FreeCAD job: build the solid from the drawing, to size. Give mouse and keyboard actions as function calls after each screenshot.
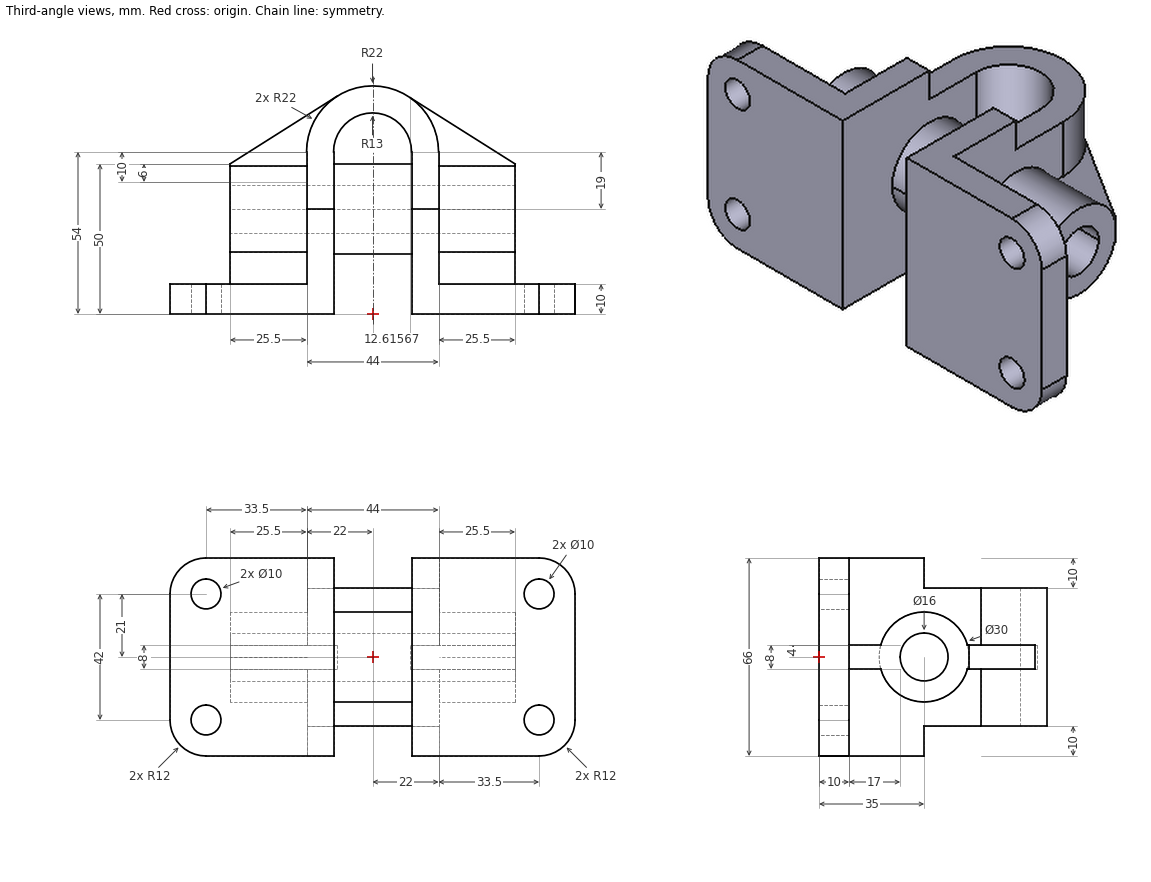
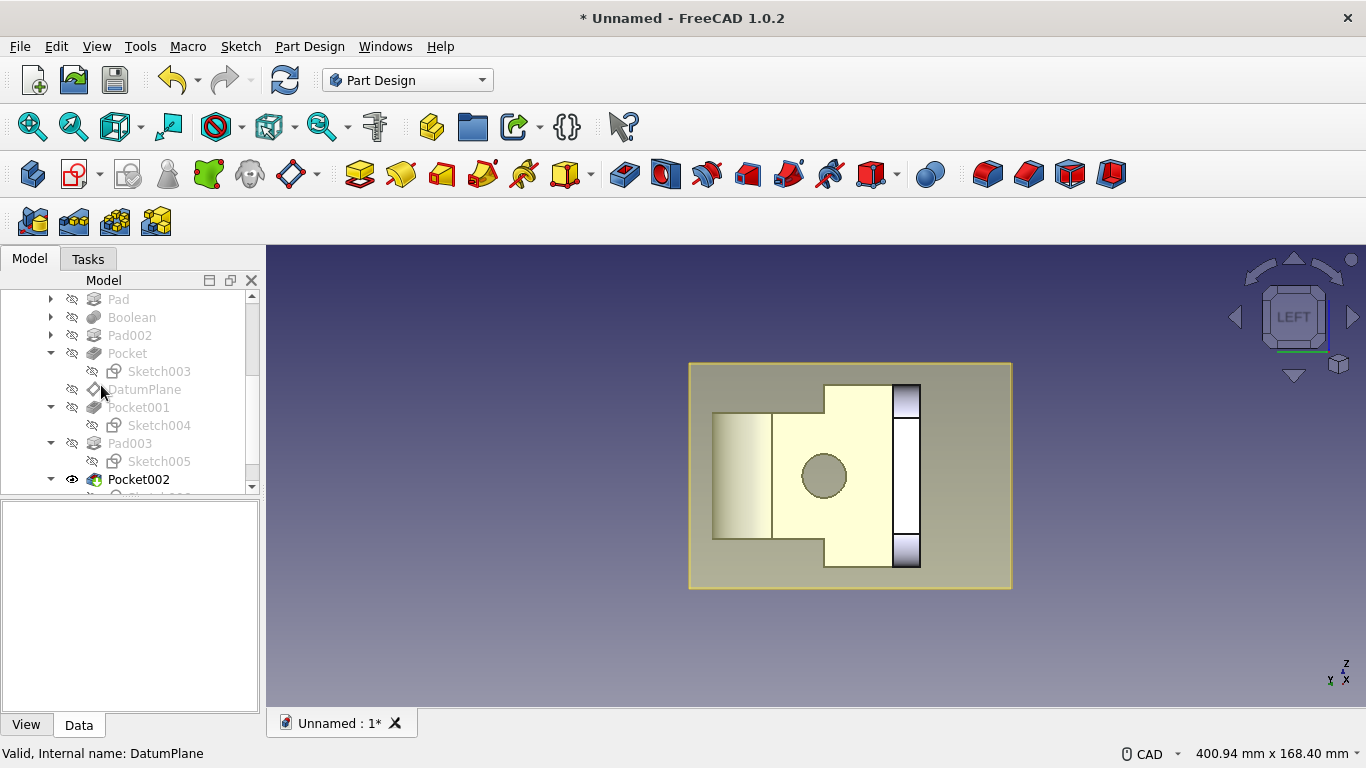
scroll(141, 385, up, 15)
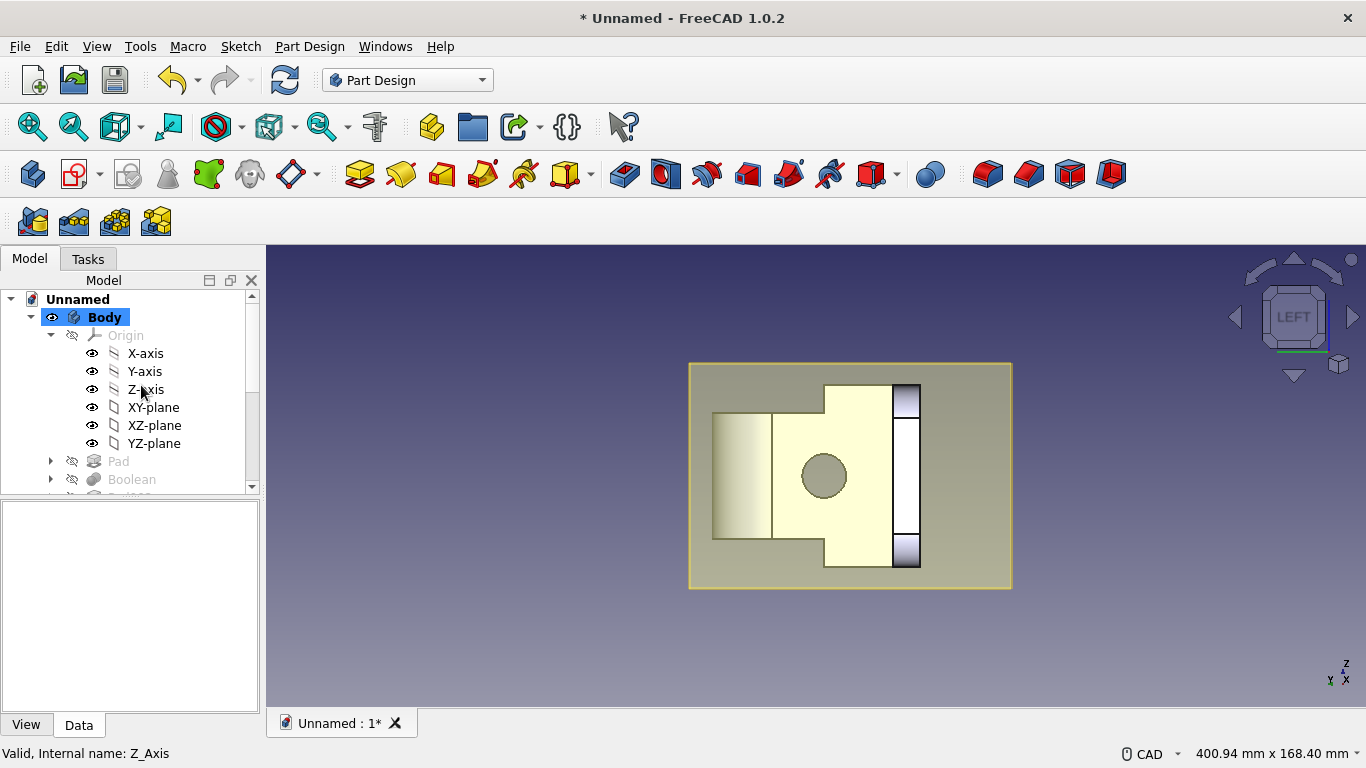
scroll(101, 385, down, 6)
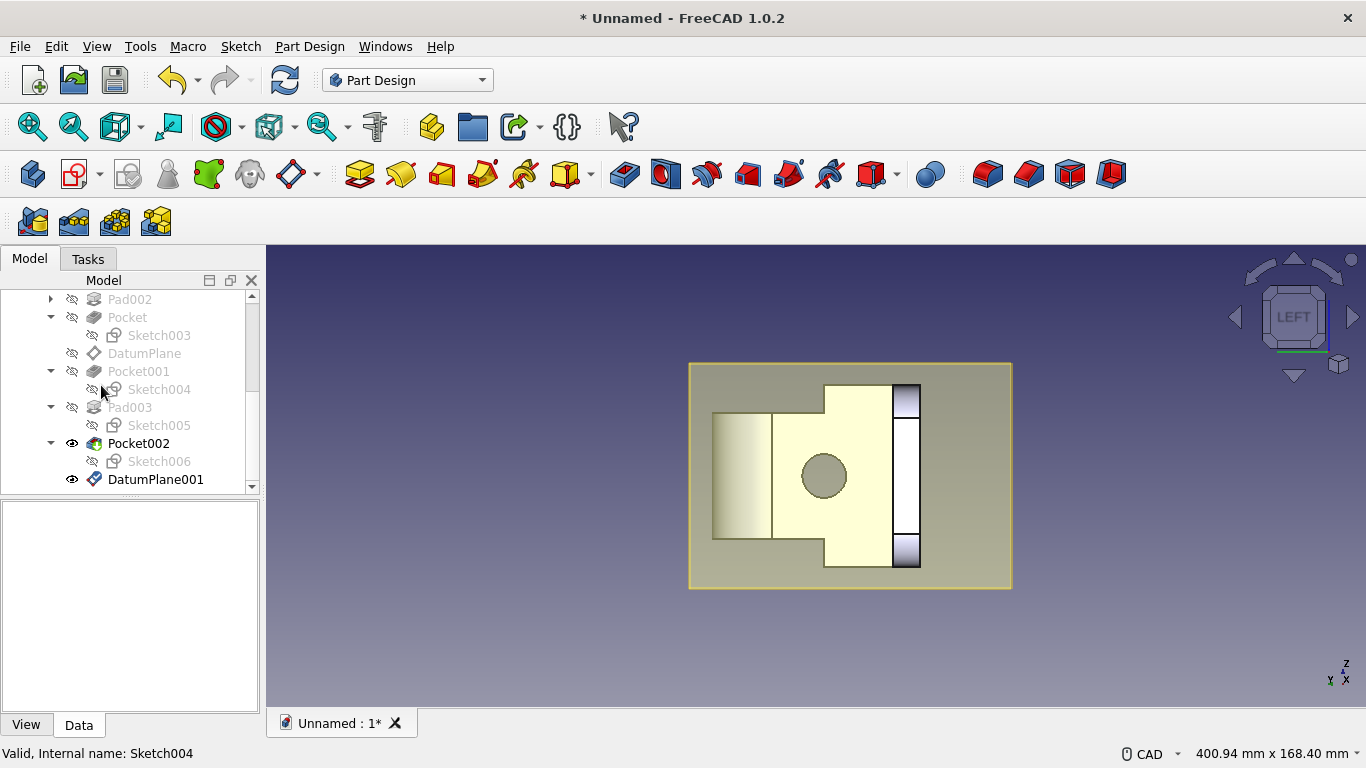
click(117, 479)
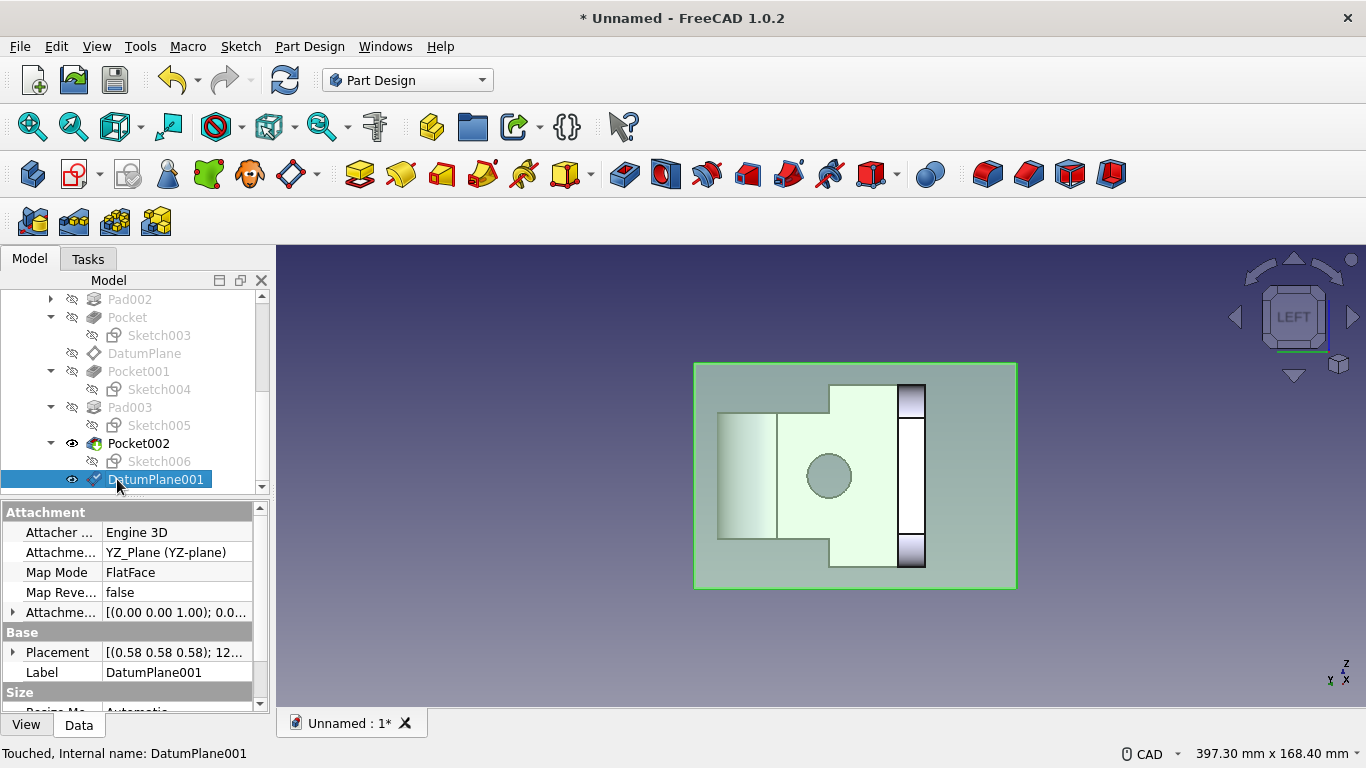
click(74, 174)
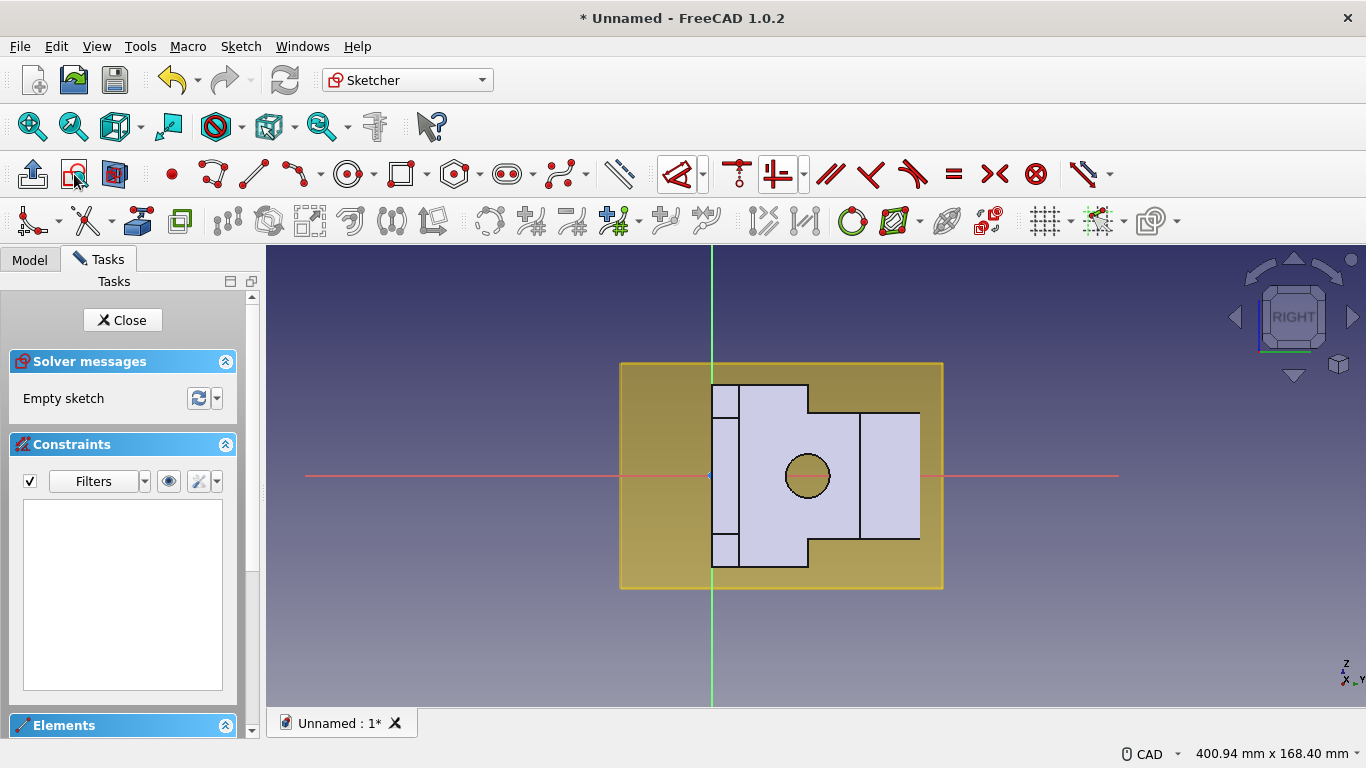
click(115, 174)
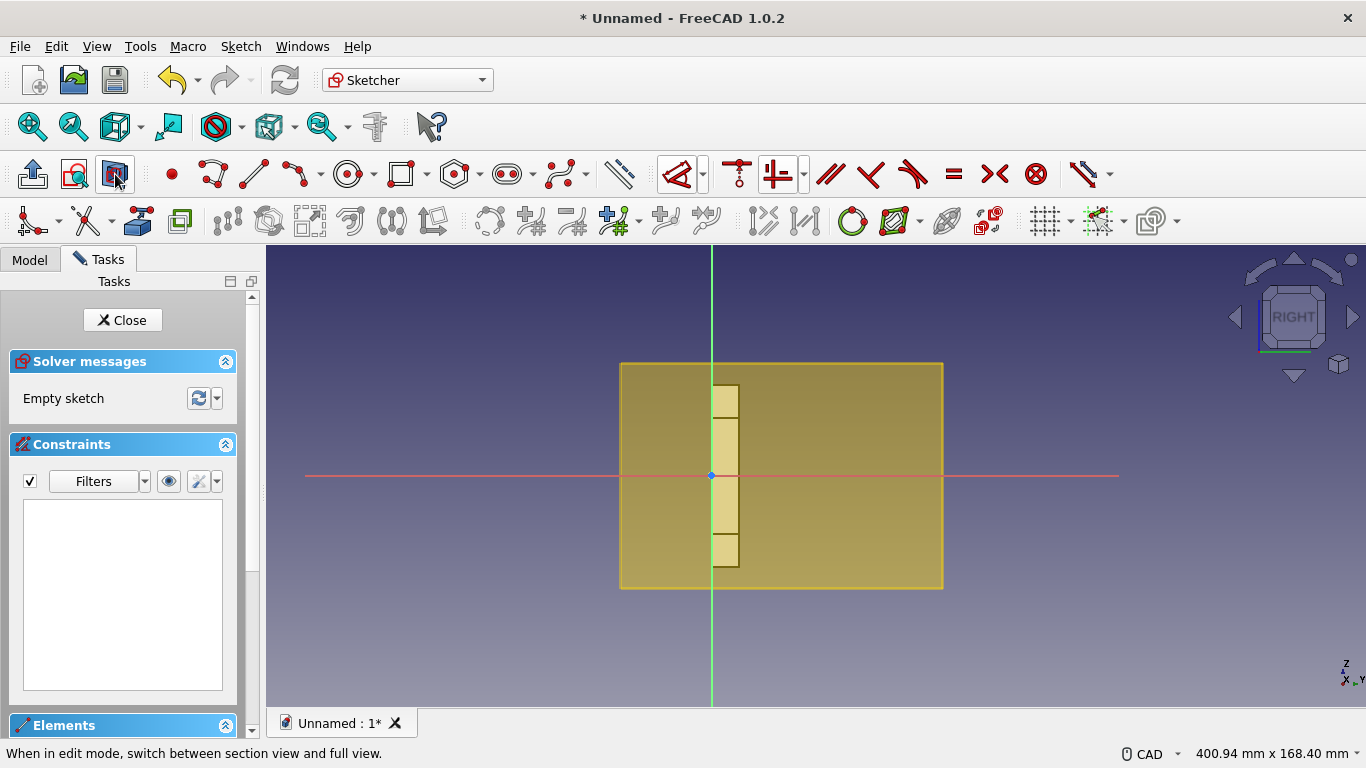
scroll(794, 476, up, 6)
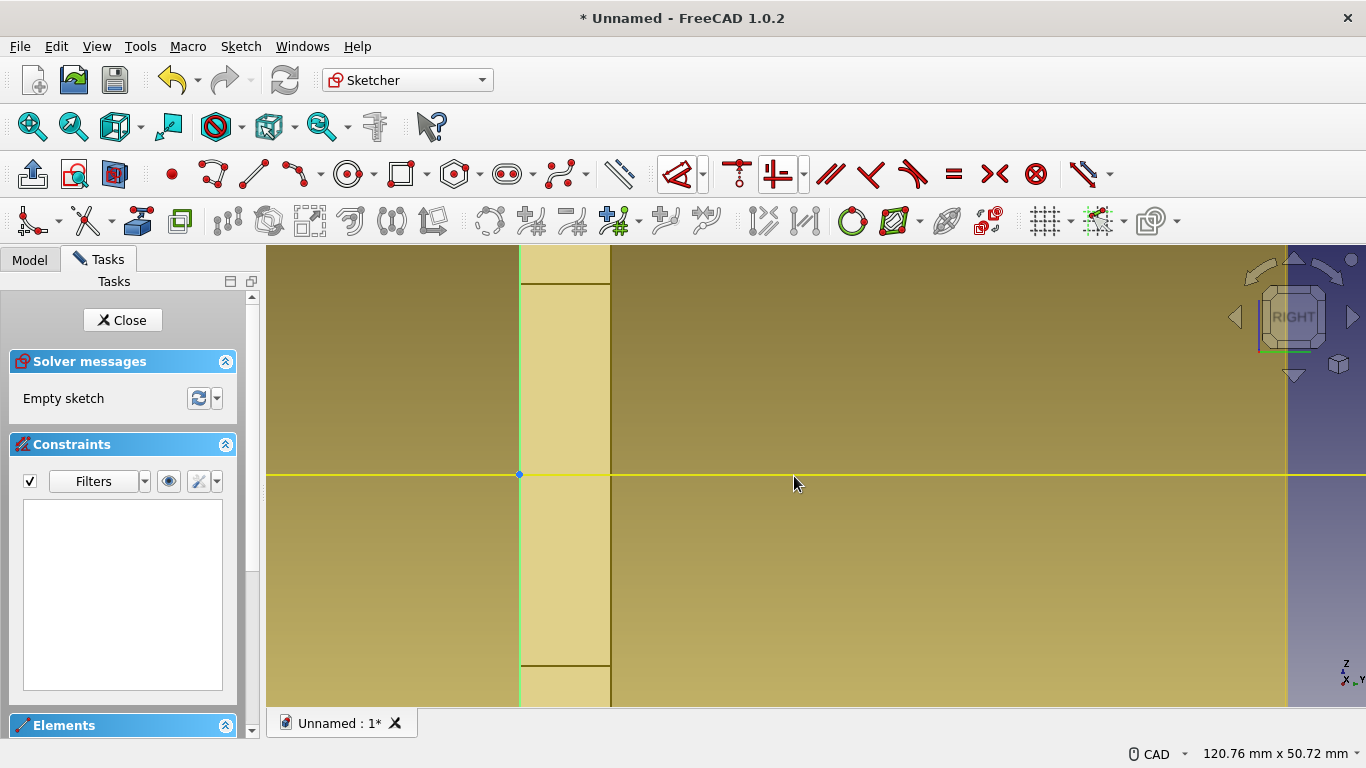
click(348, 174)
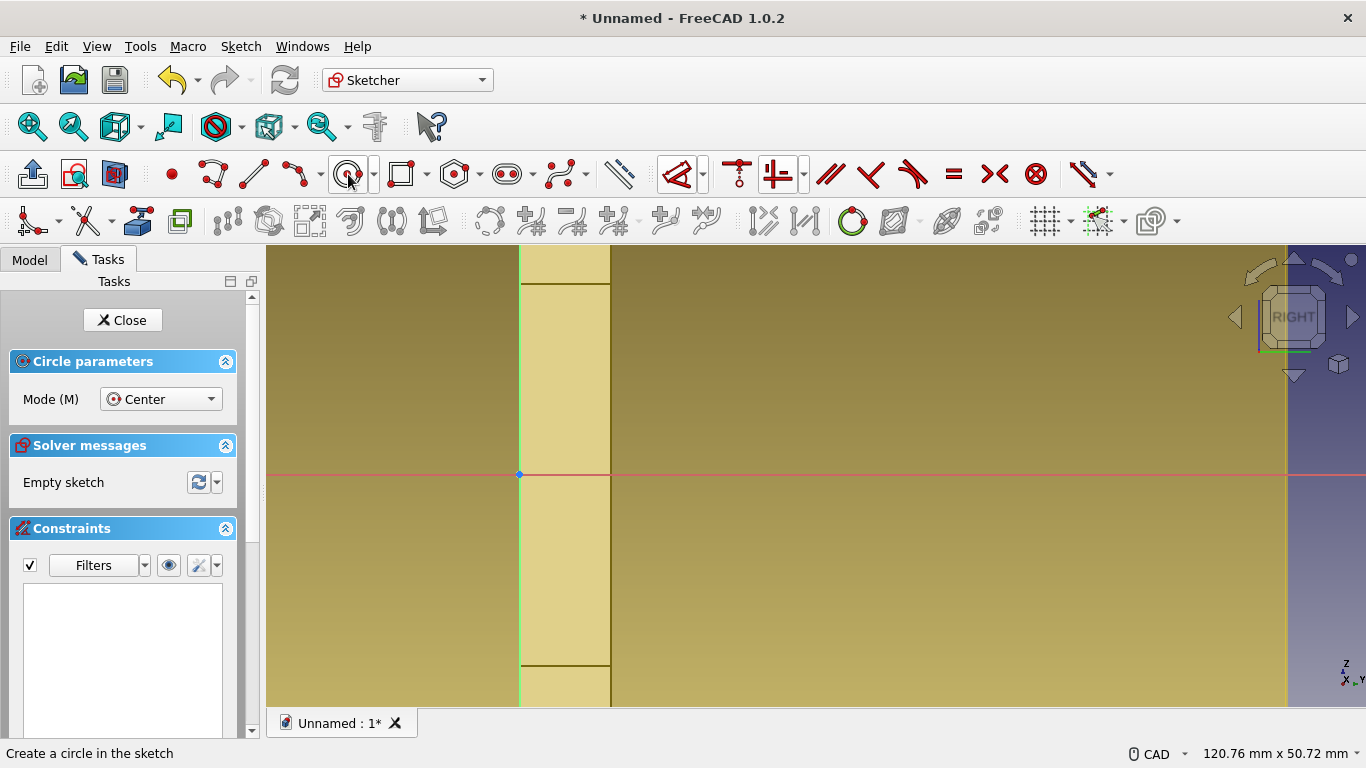
click(839, 475)
move(935, 378)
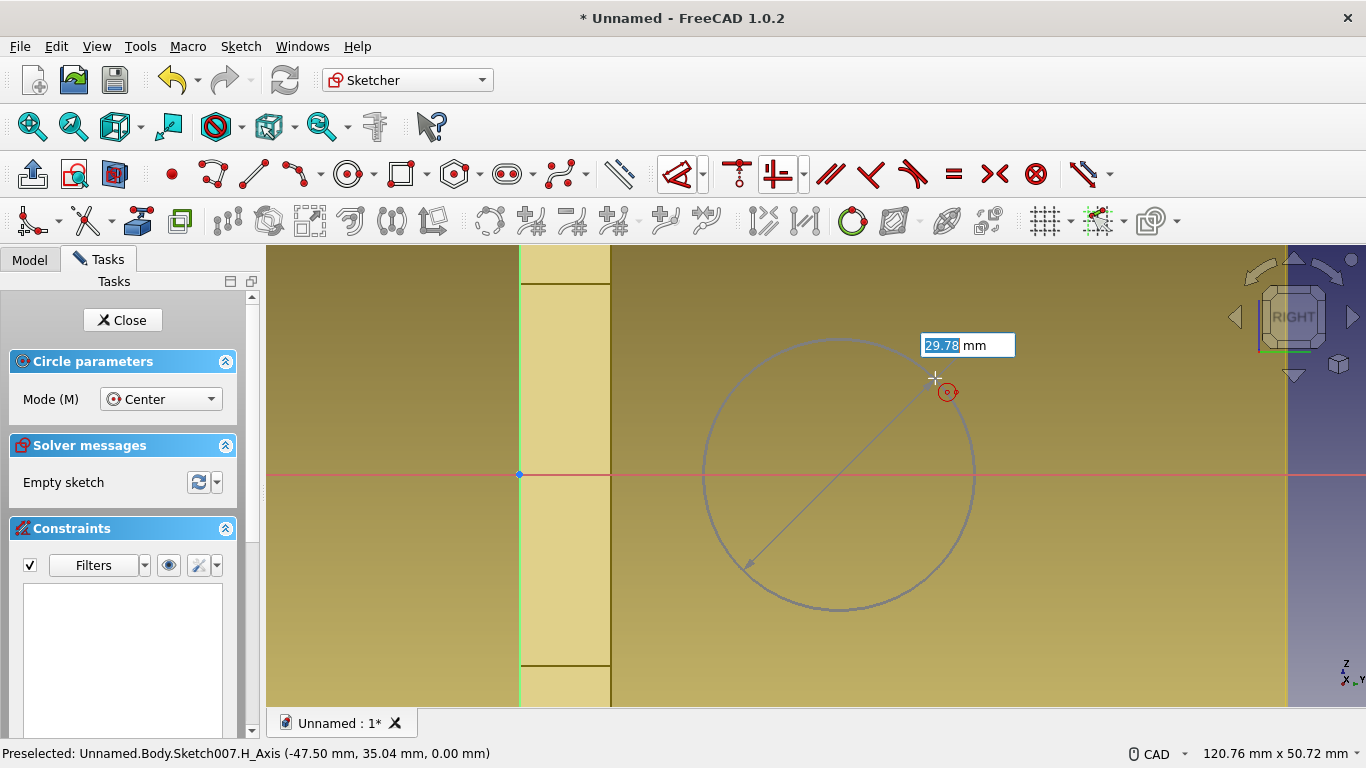
text(30)
key(Return)